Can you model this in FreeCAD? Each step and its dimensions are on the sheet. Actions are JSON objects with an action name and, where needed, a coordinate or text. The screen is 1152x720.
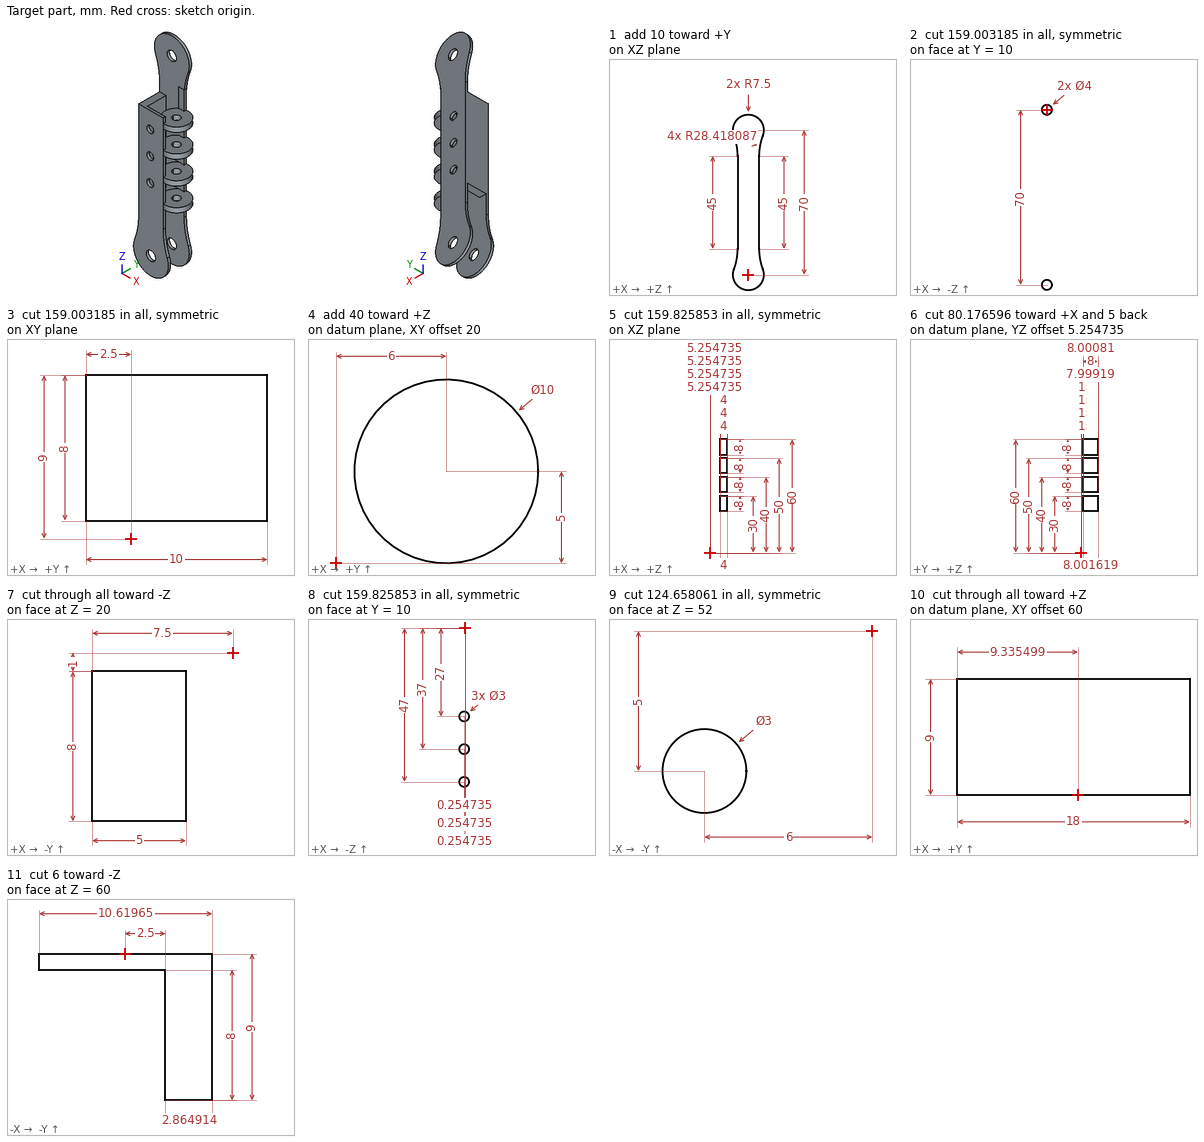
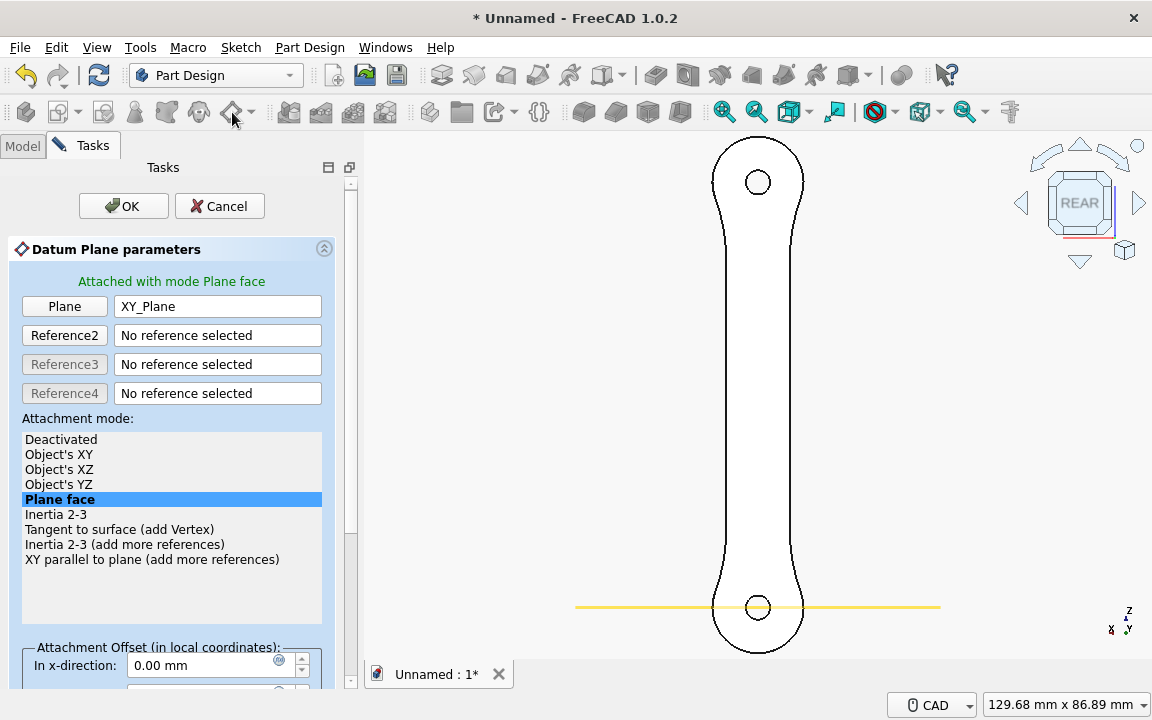
{"action": "scroll", "coordinate": [351, 432], "scroll_direction": "down", "scroll_amount": 2}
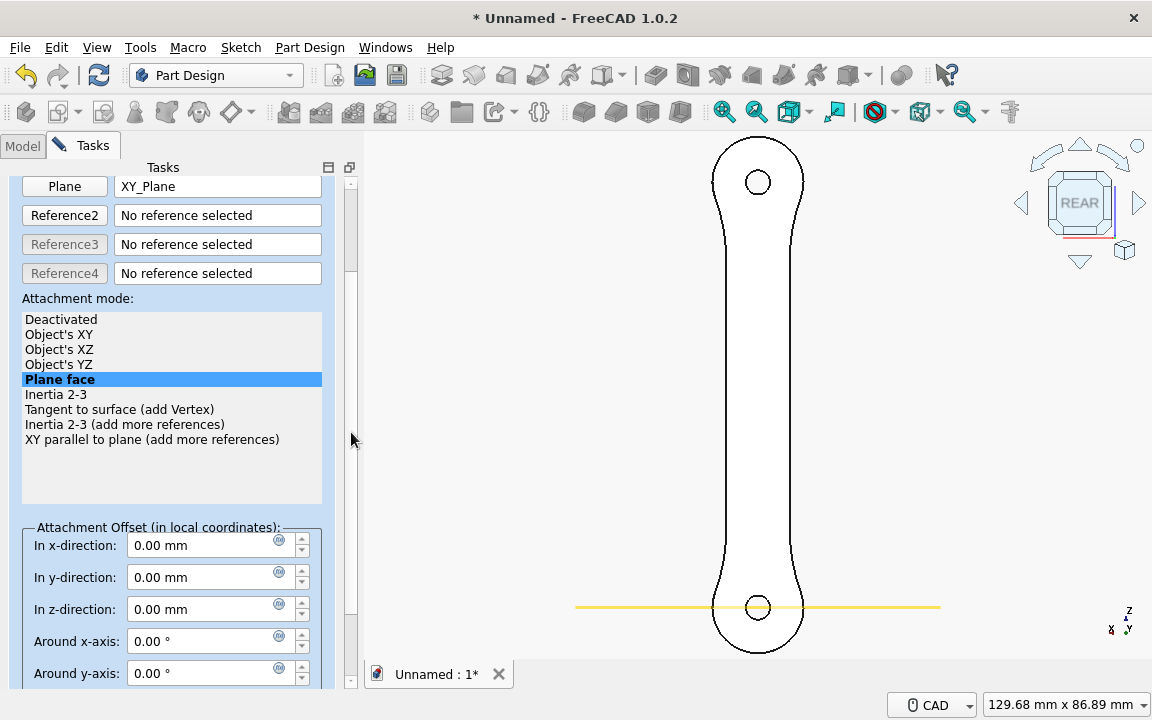
{"action": "triple_click", "coordinate": [210, 609]}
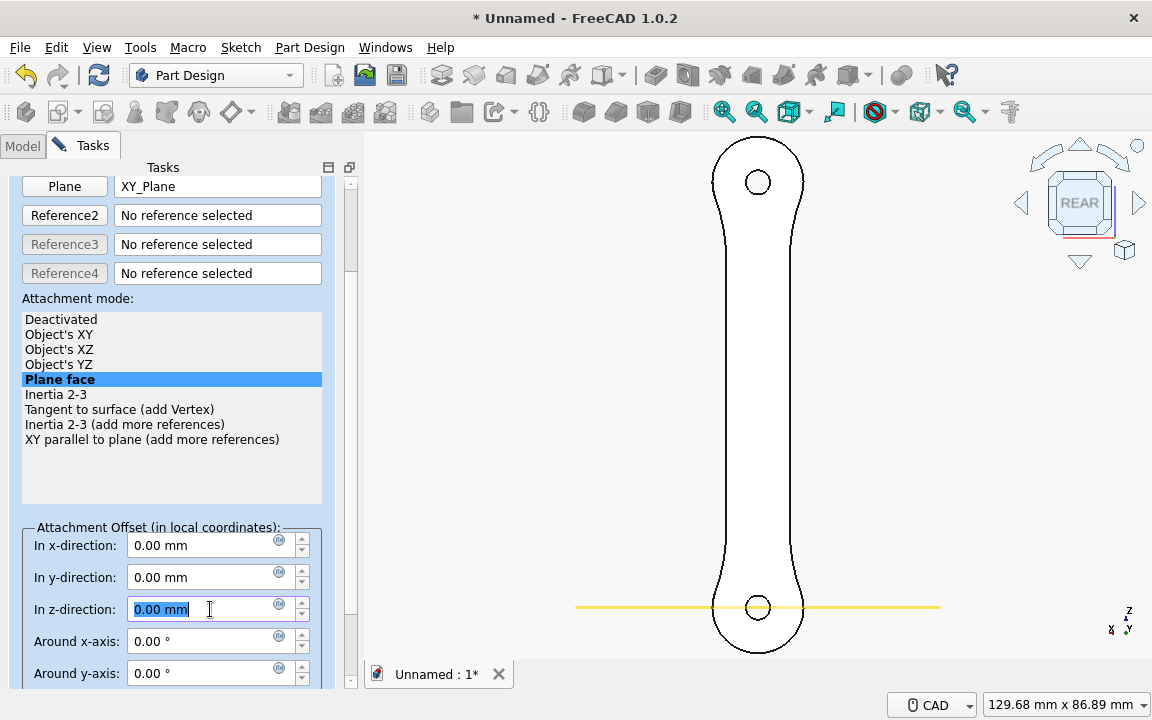
{"action": "type", "text": "20"}
{"action": "key", "text": "Tab"}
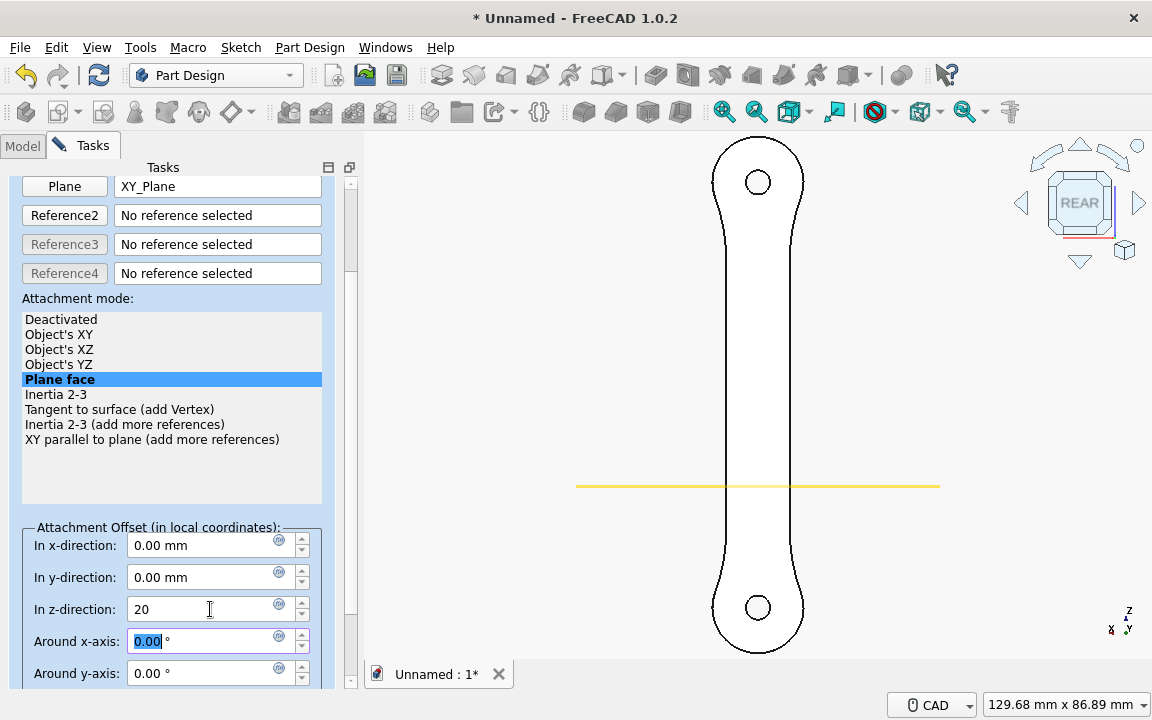
{"action": "scroll", "coordinate": [351, 432], "scroll_direction": "up", "scroll_amount": 3}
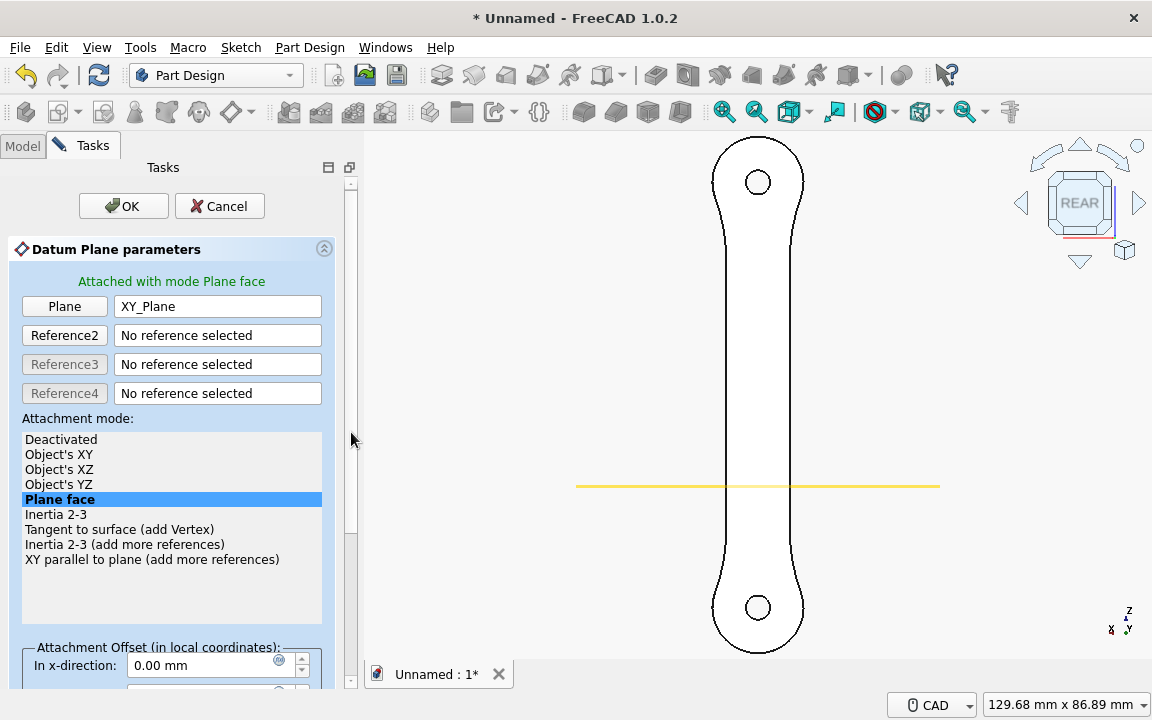
{"action": "left_click", "coordinate": [124, 206]}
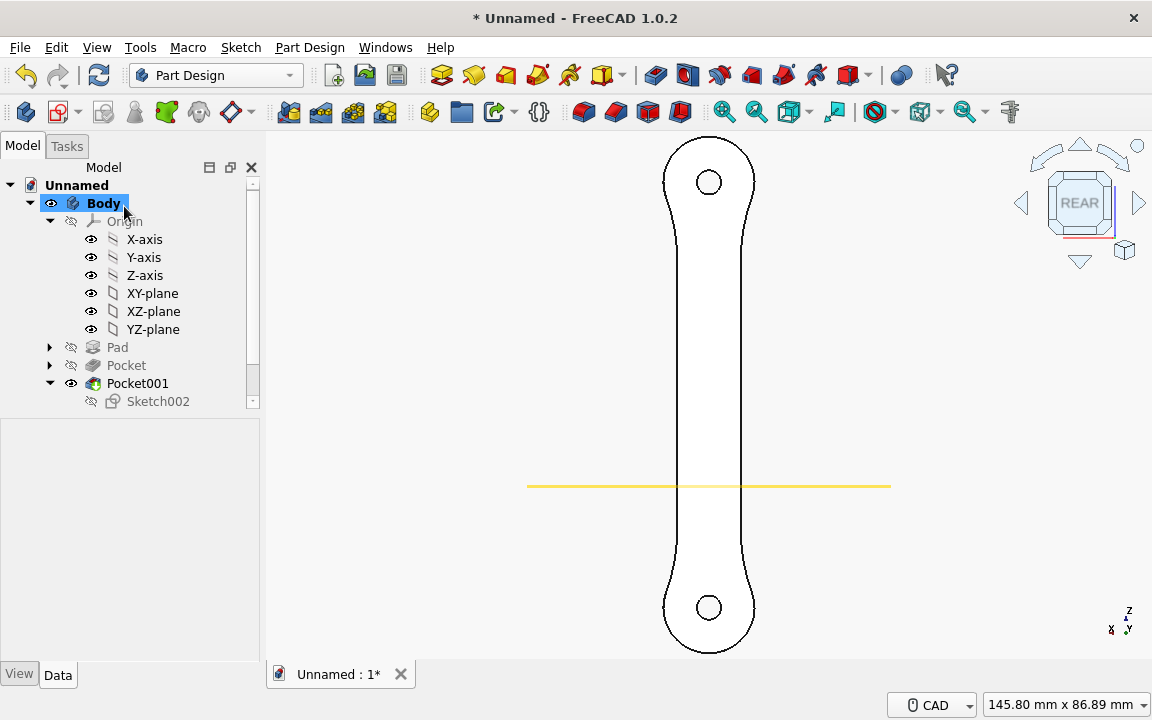
{"action": "scroll", "coordinate": [100, 289], "scroll_direction": "down", "scroll_amount": 3}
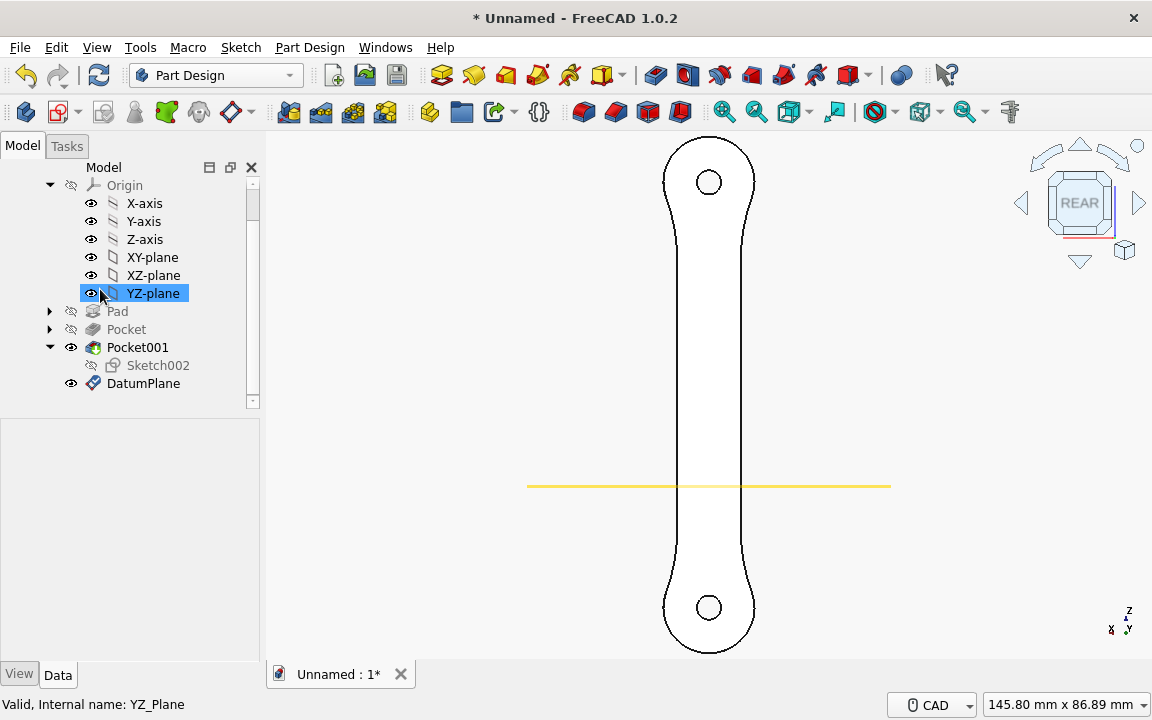
{"action": "left_click", "coordinate": [116, 383]}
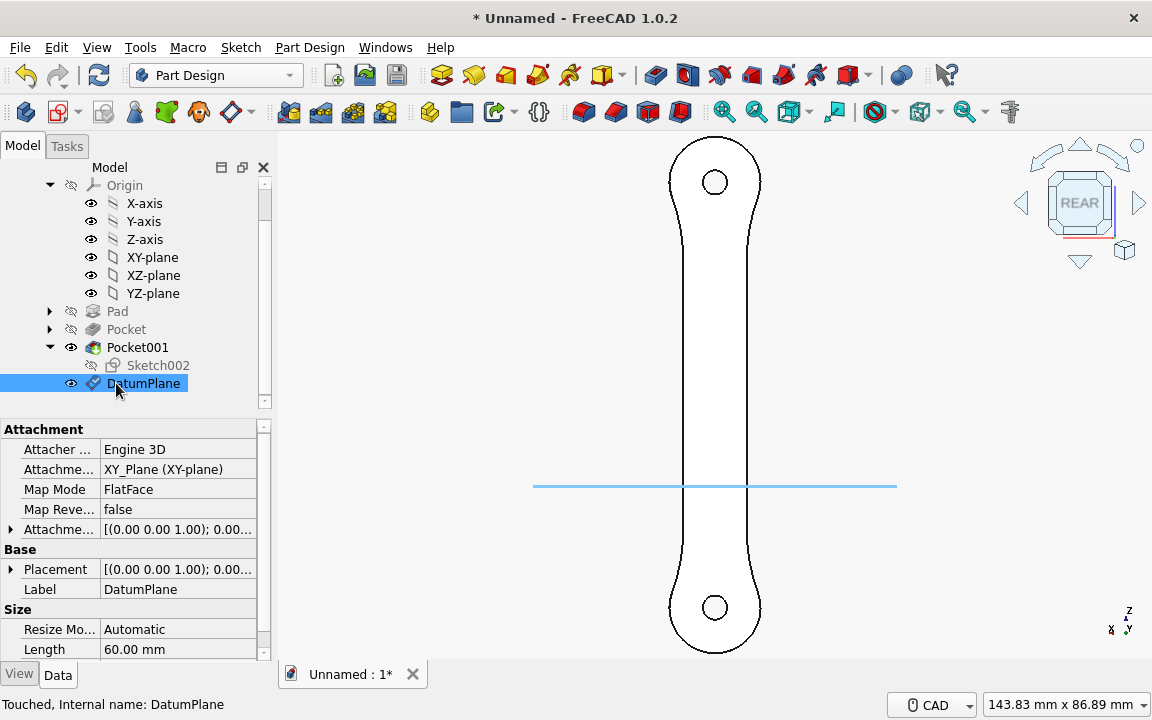
{"action": "left_click", "coordinate": [58, 112]}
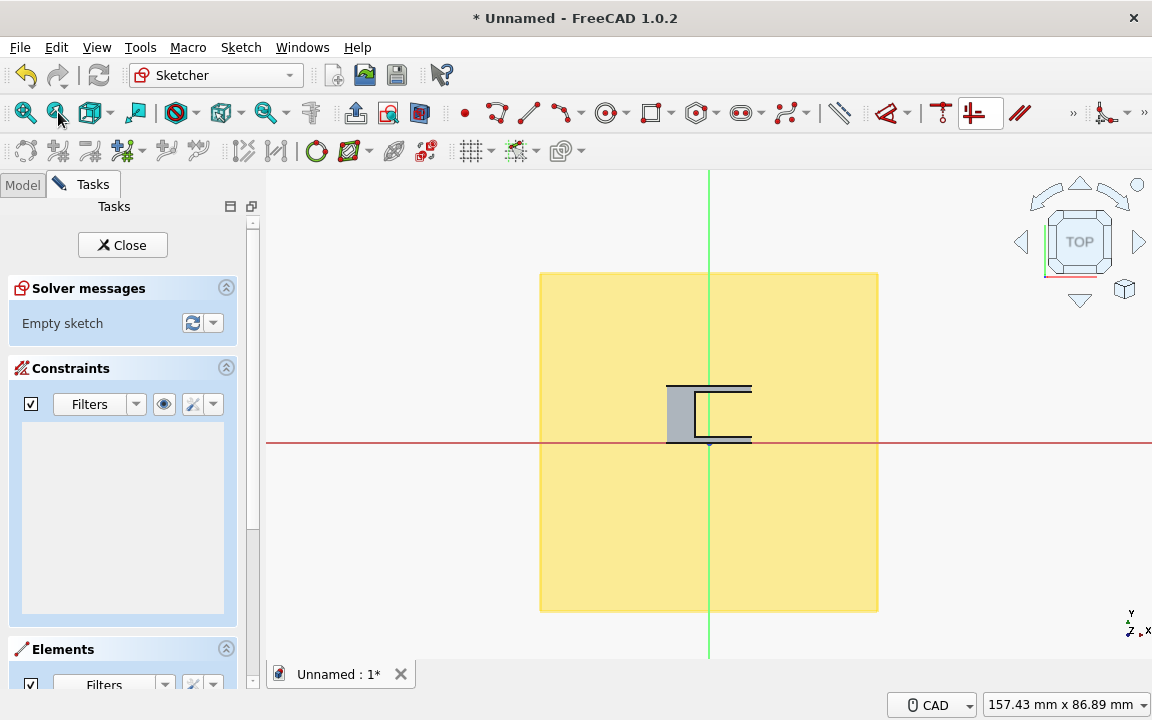
{"action": "left_click", "coordinate": [420, 114]}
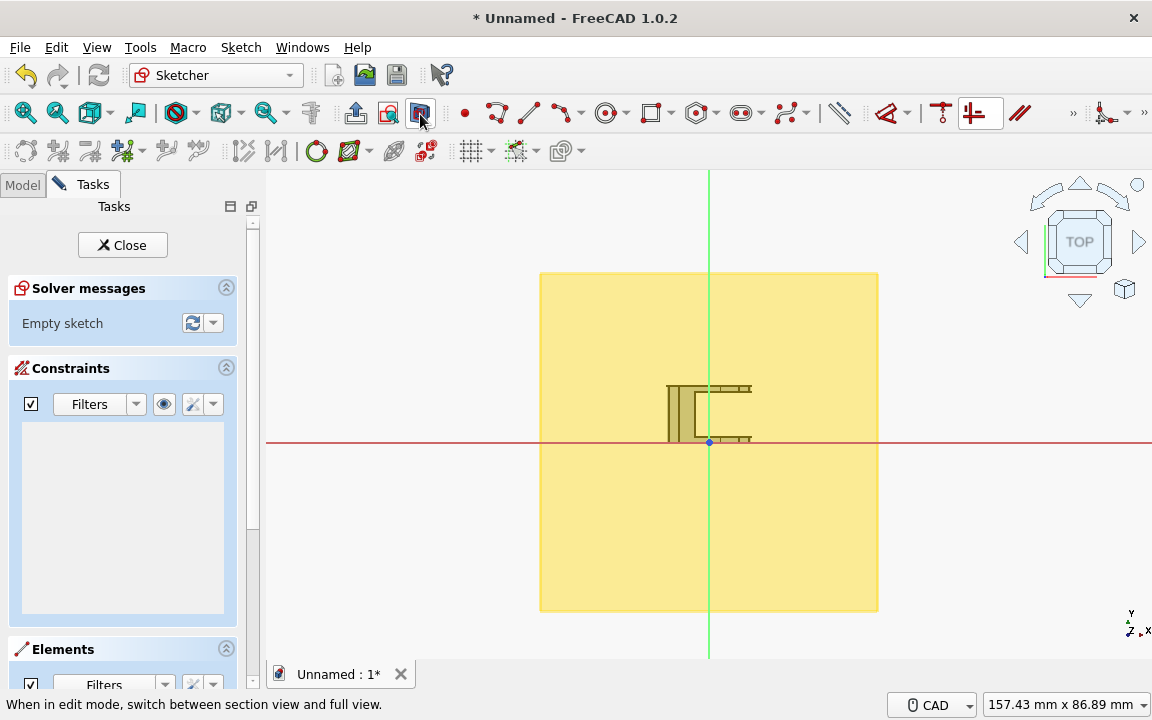
{"action": "scroll", "coordinate": [765, 414], "scroll_direction": "up", "scroll_amount": 8}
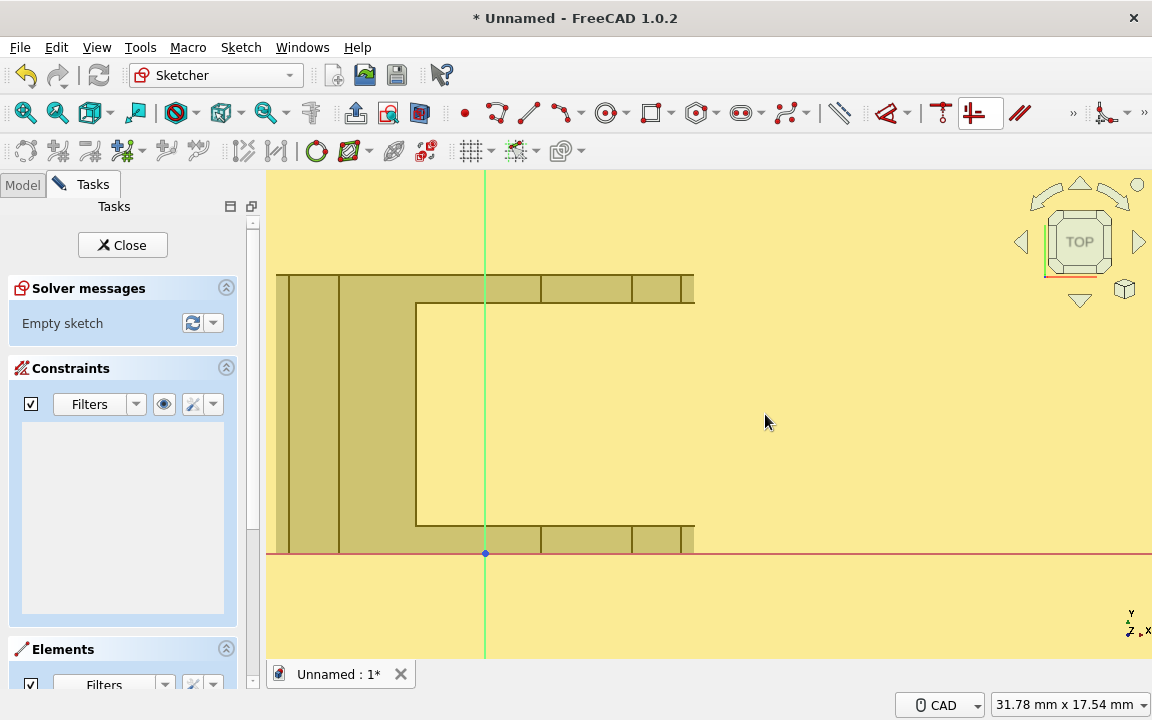
{"action": "left_click", "coordinate": [606, 114]}